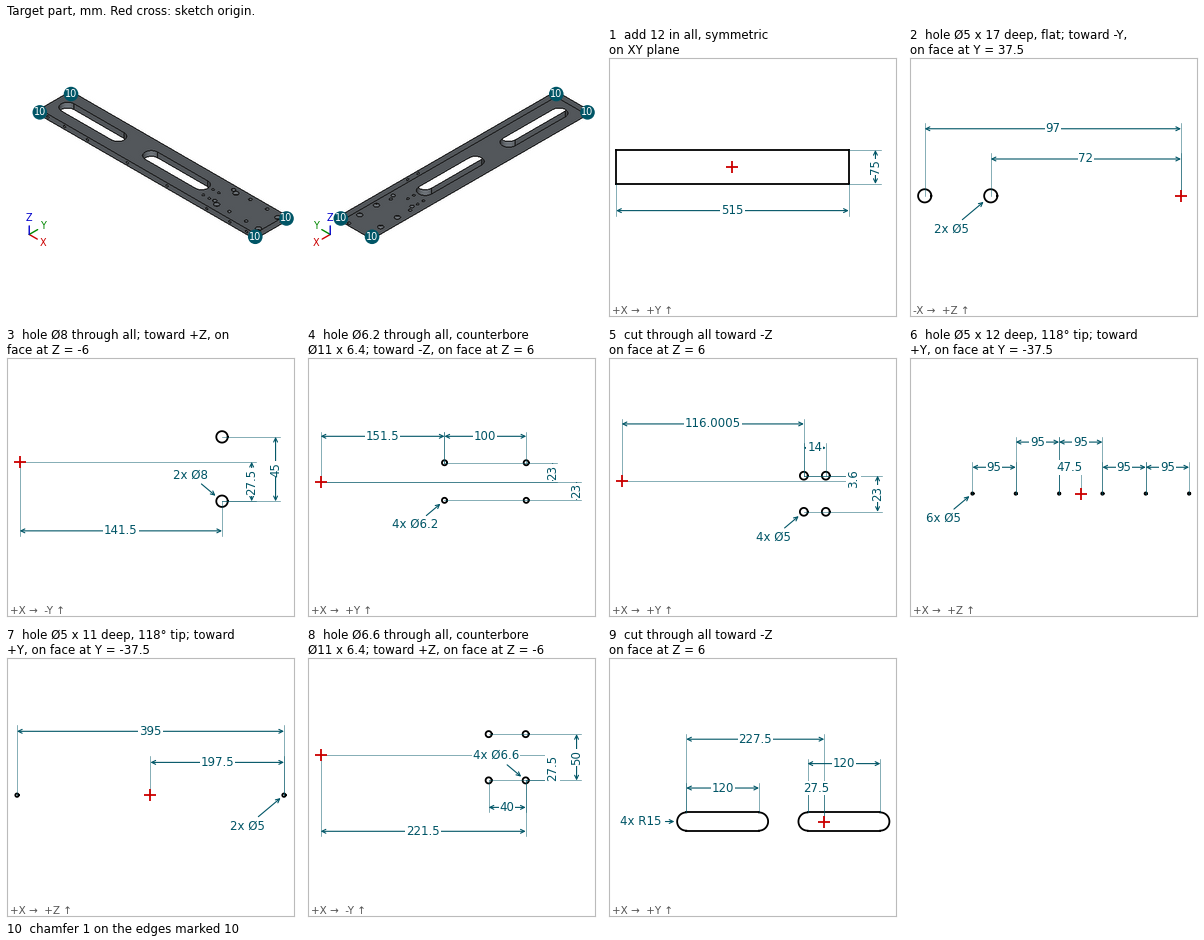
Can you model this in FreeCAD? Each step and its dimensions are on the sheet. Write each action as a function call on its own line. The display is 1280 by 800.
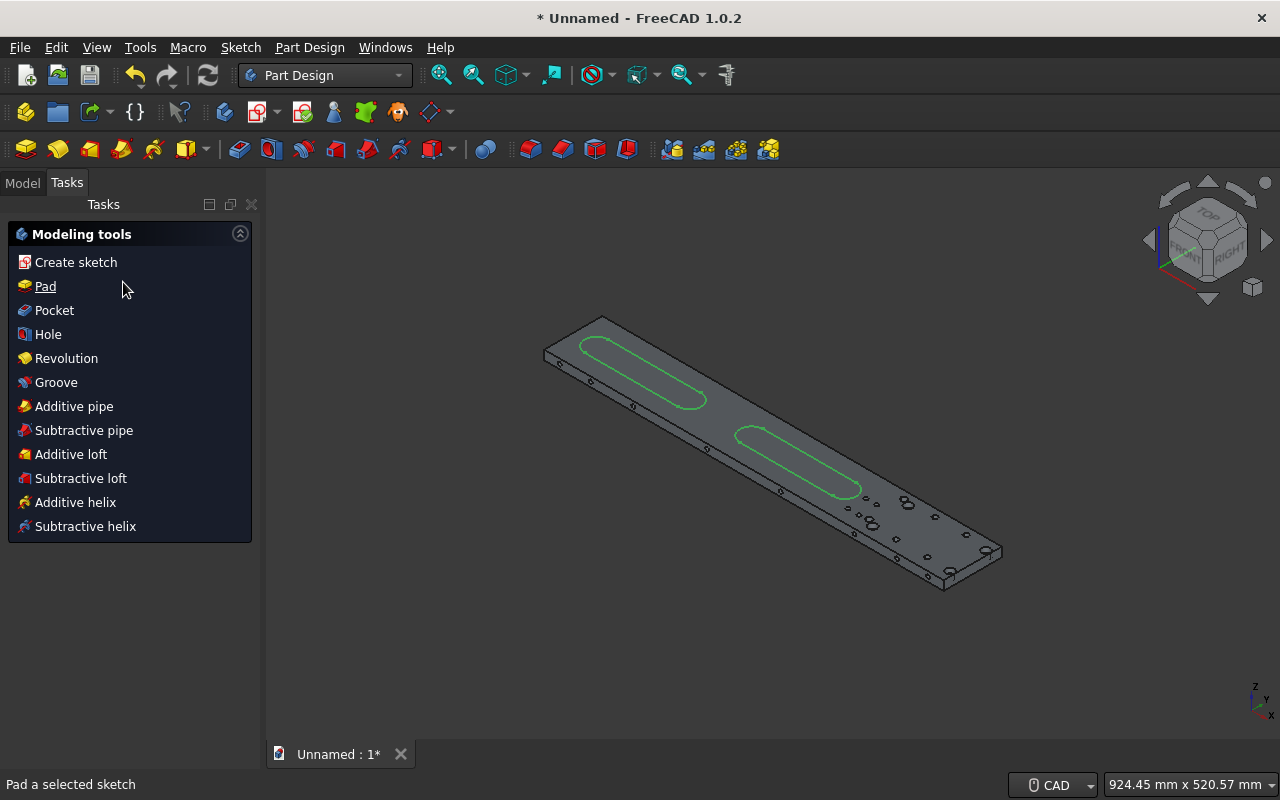
click(240, 150)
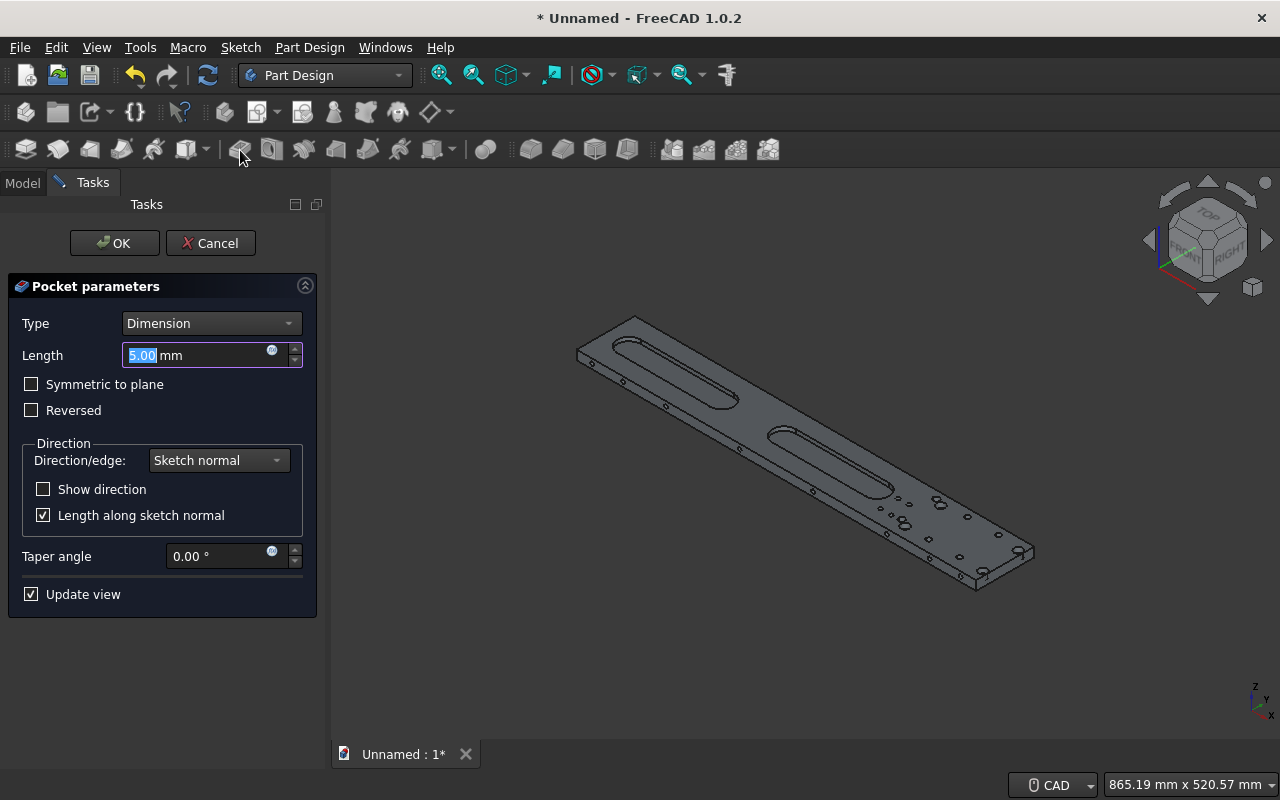
click(212, 324)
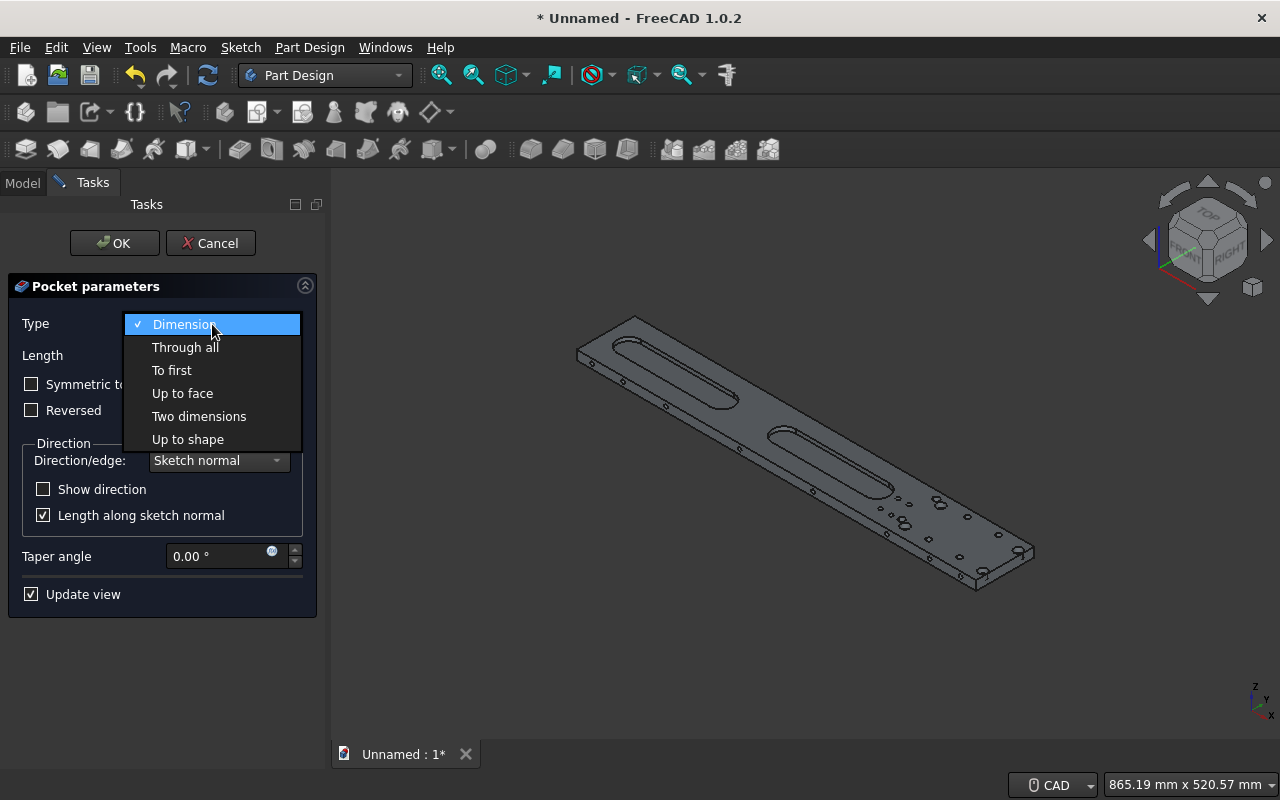
click(212, 348)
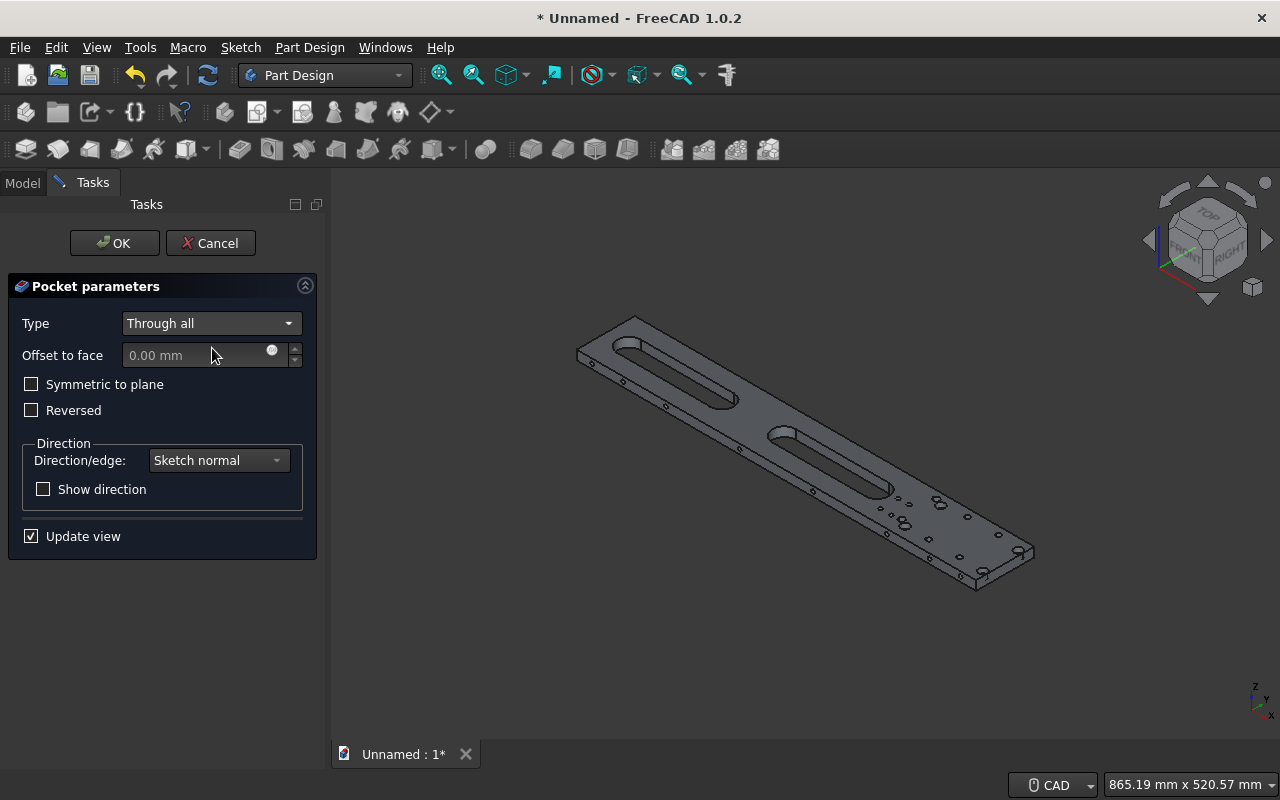
click(115, 243)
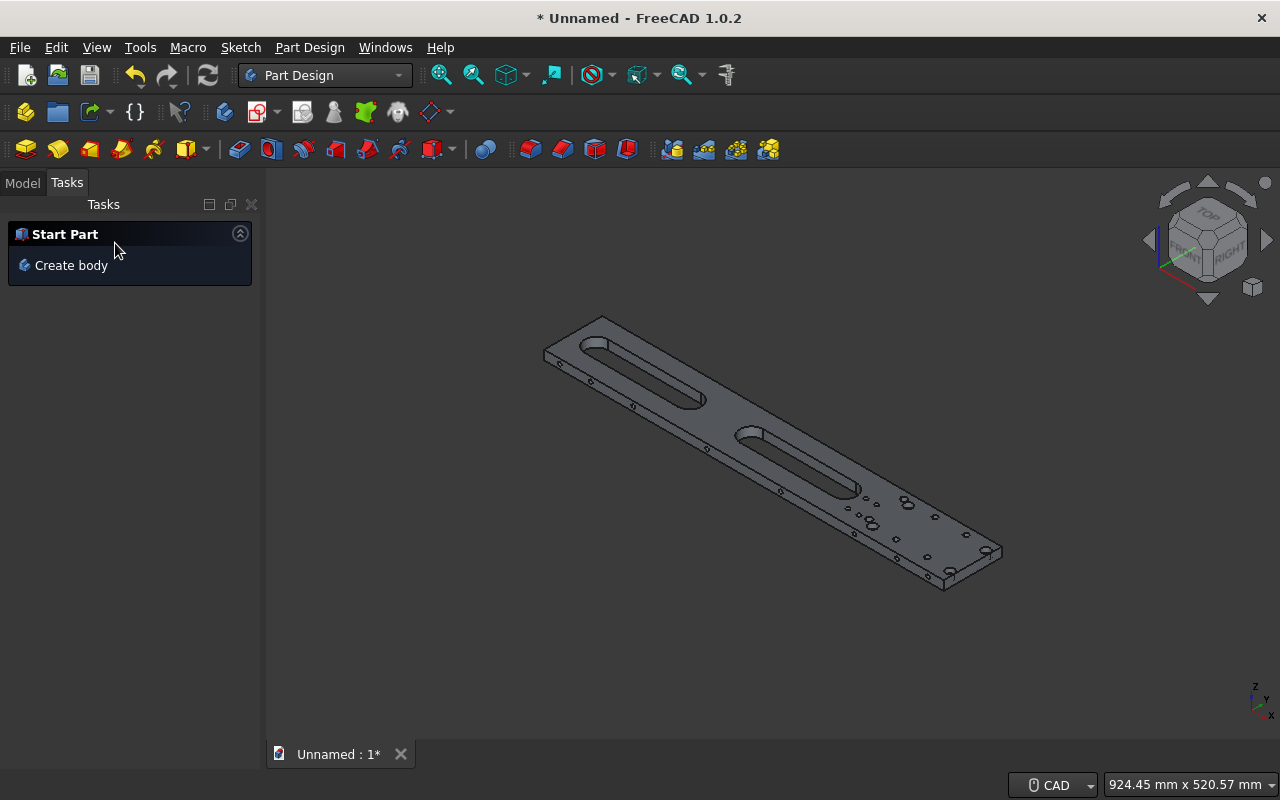
click(944, 586)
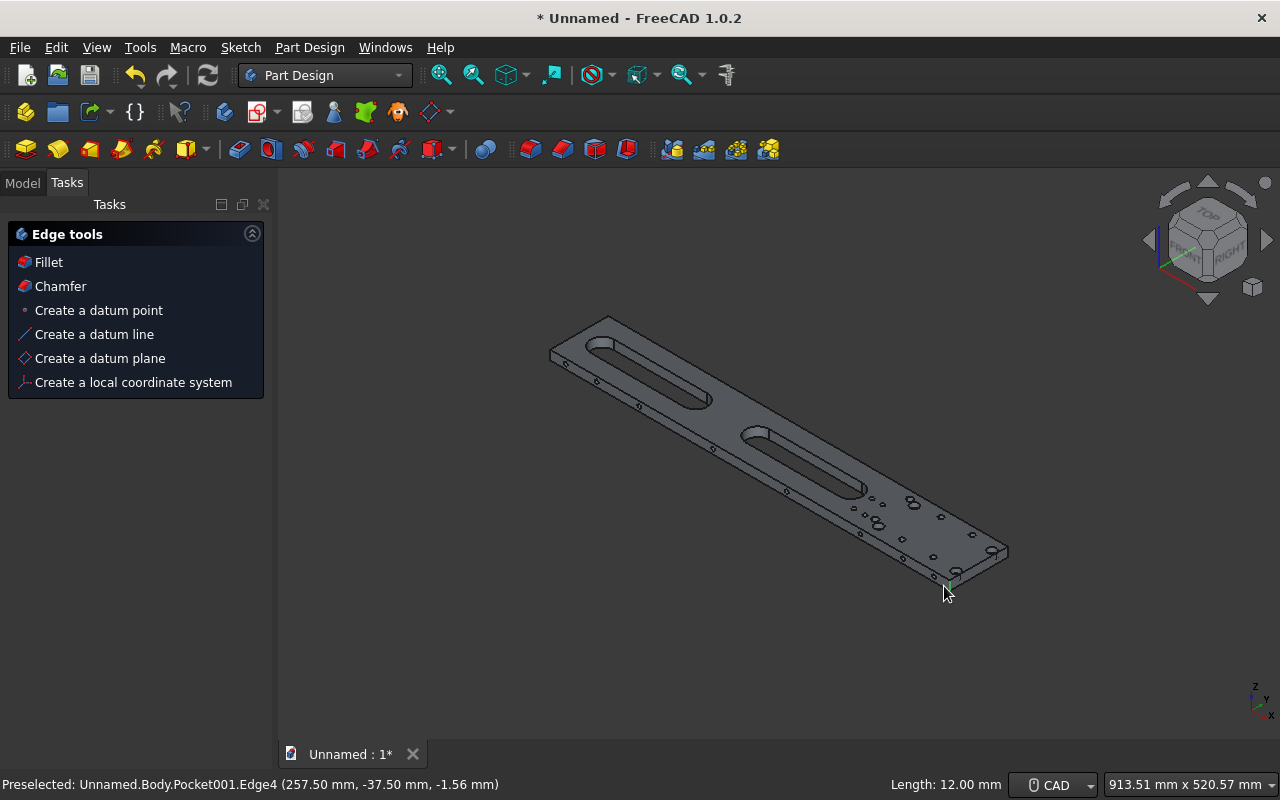
scroll(550, 354, up, 6)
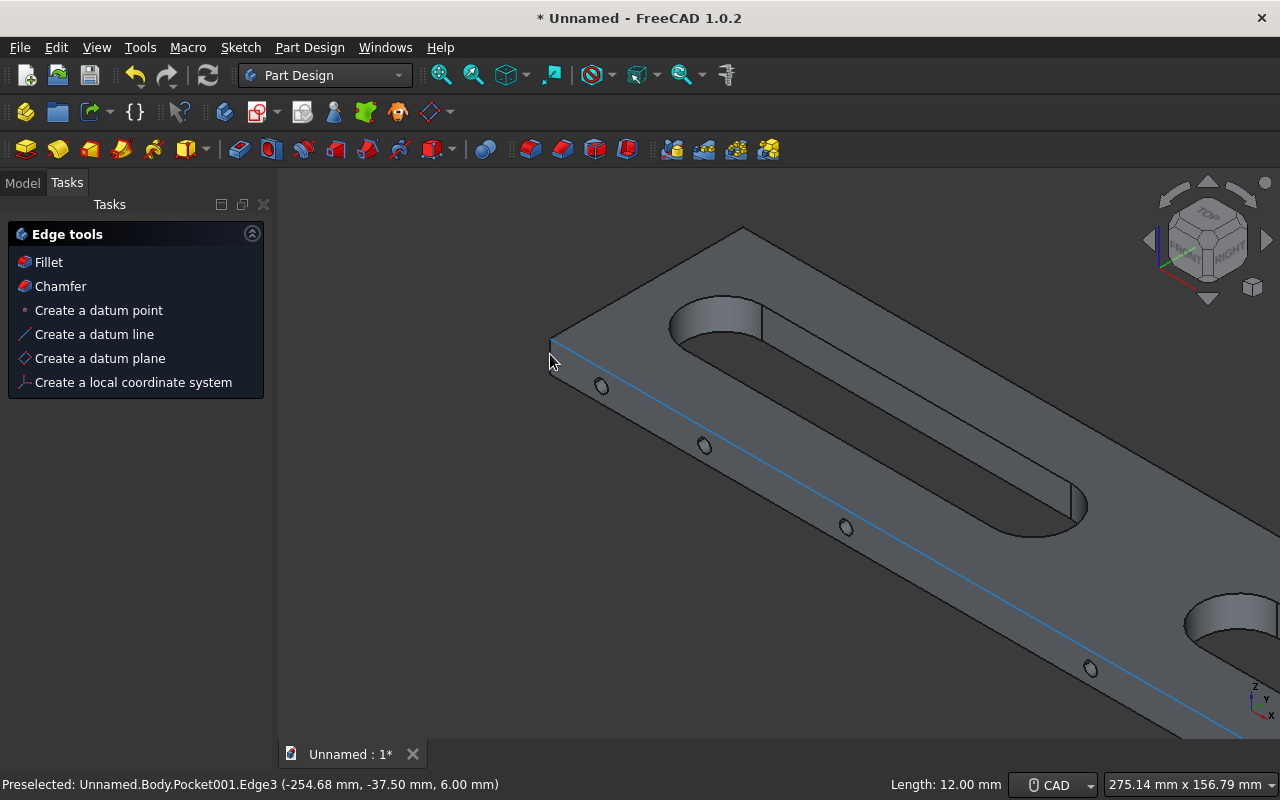
key(v)
key(f)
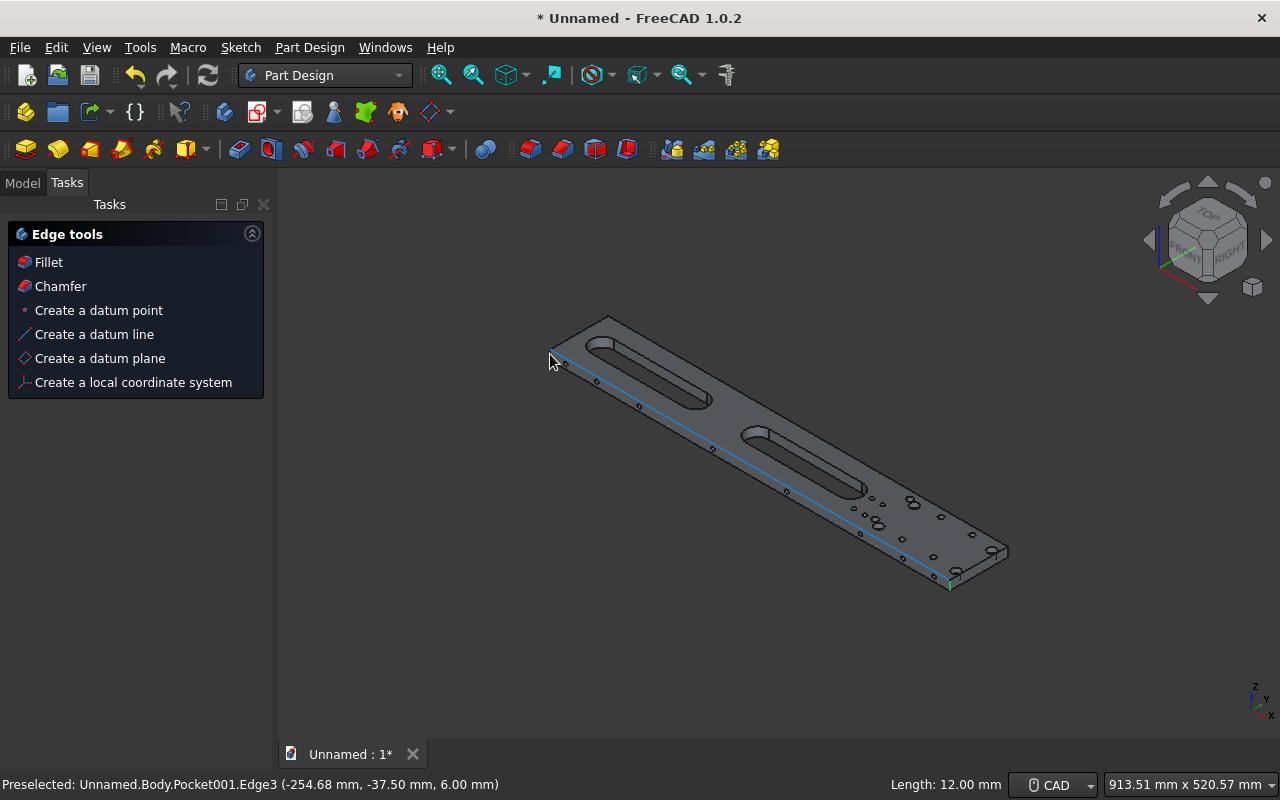
key(2)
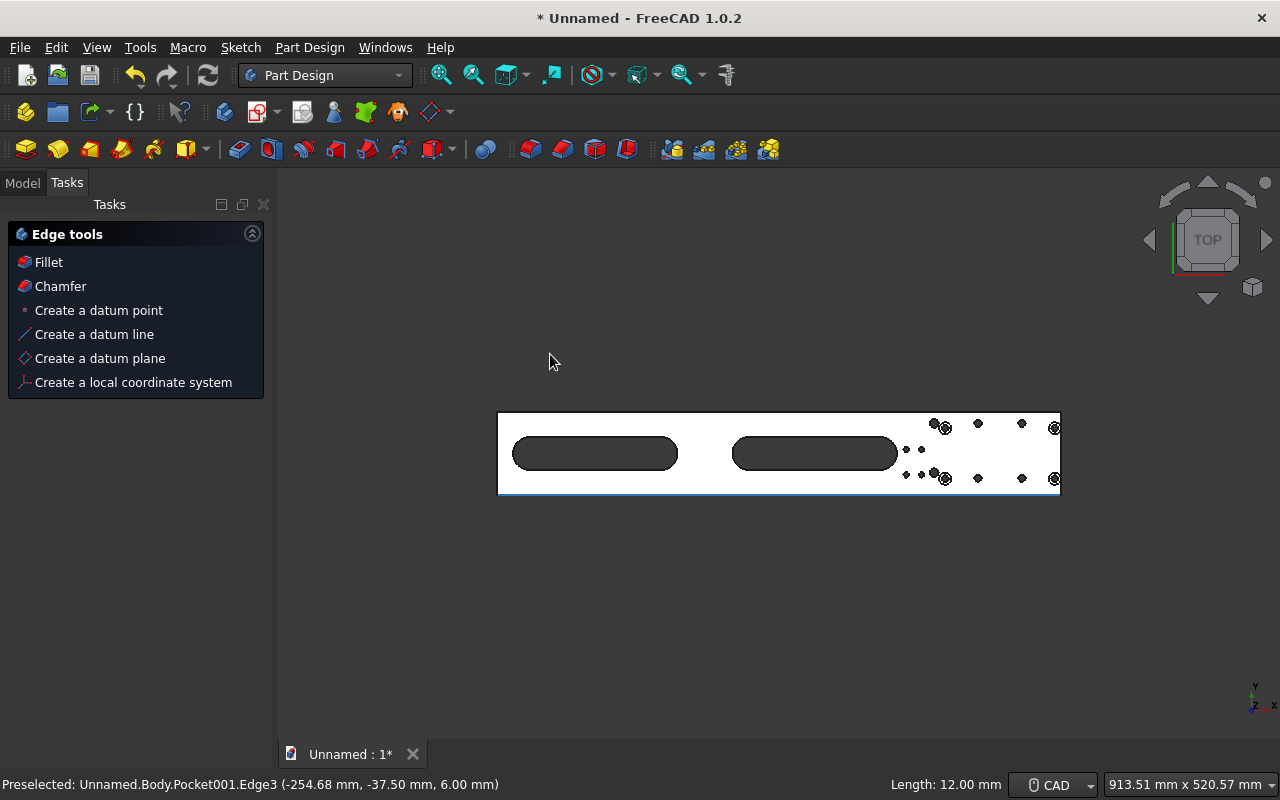
scroll(497, 494, up, 6)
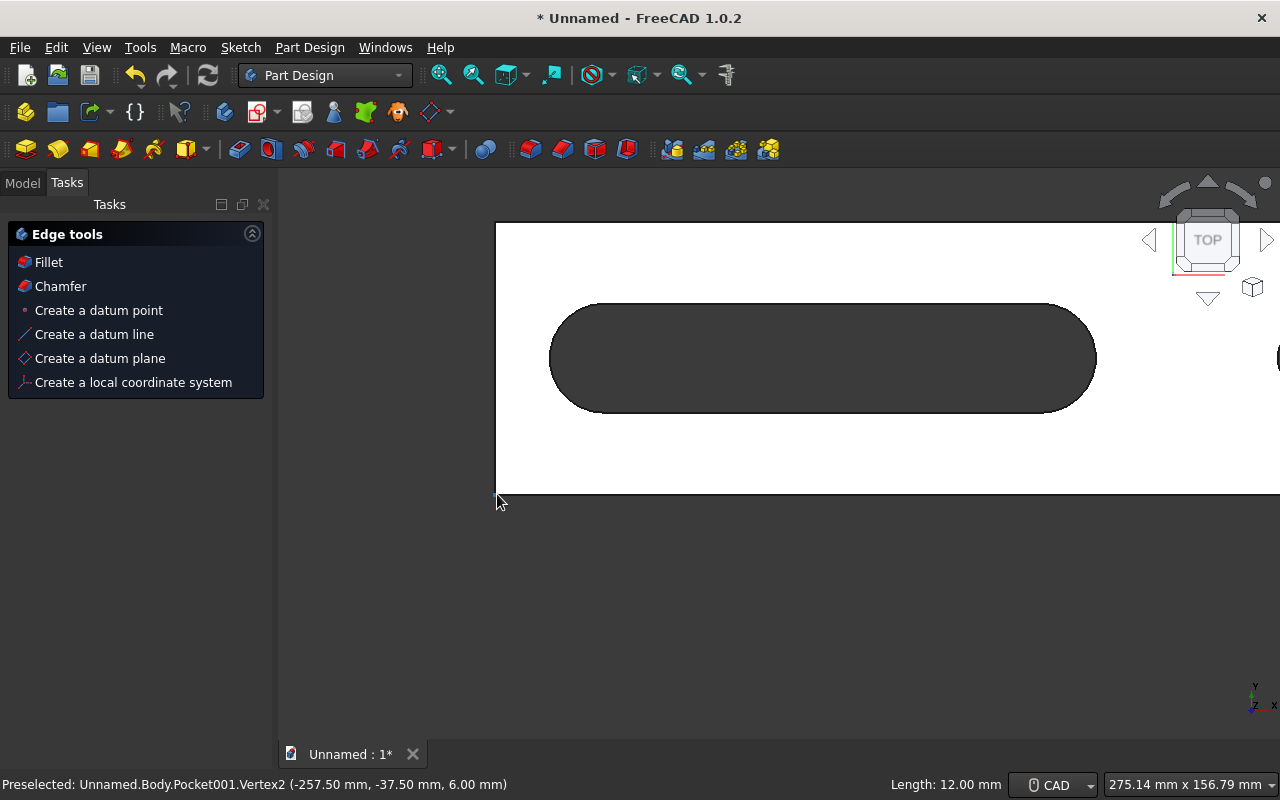
click(442, 76)